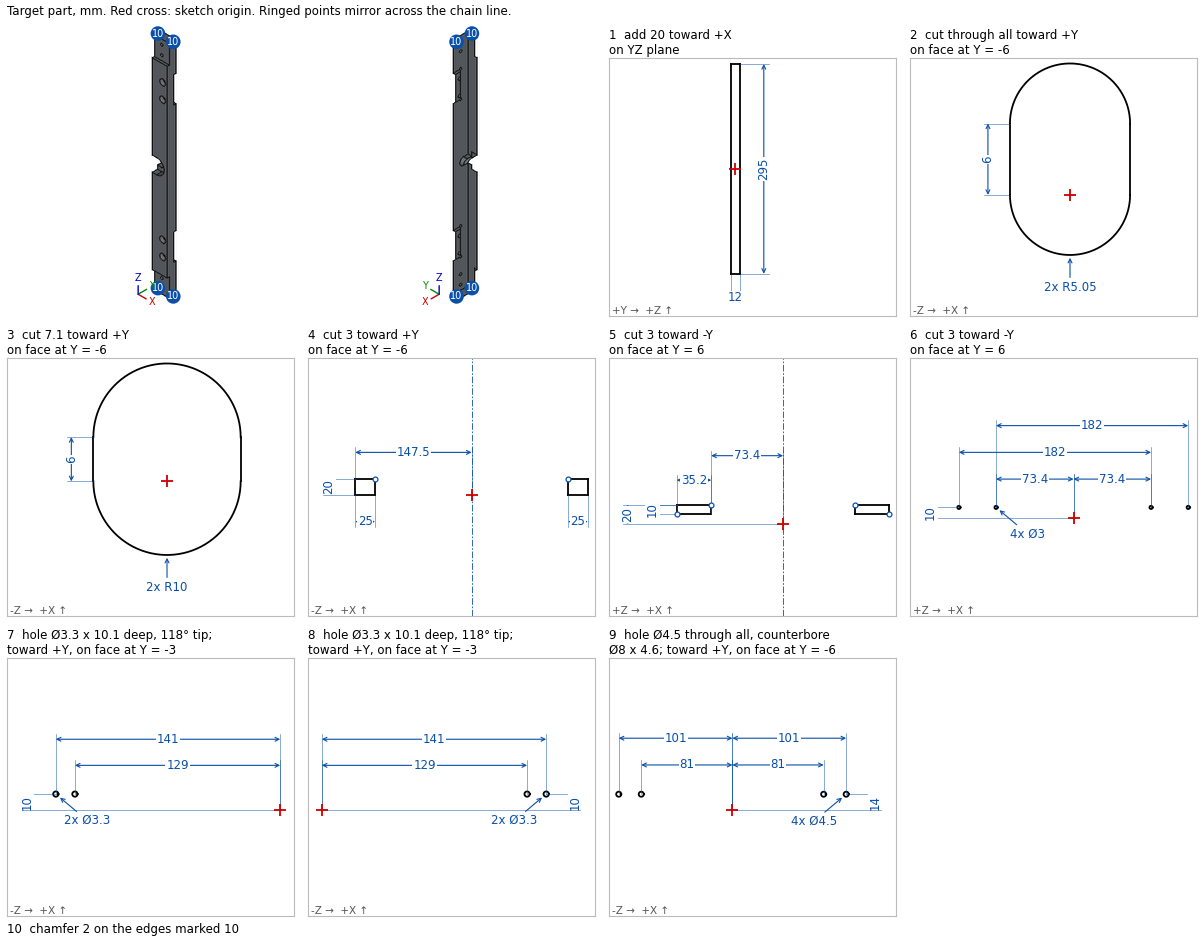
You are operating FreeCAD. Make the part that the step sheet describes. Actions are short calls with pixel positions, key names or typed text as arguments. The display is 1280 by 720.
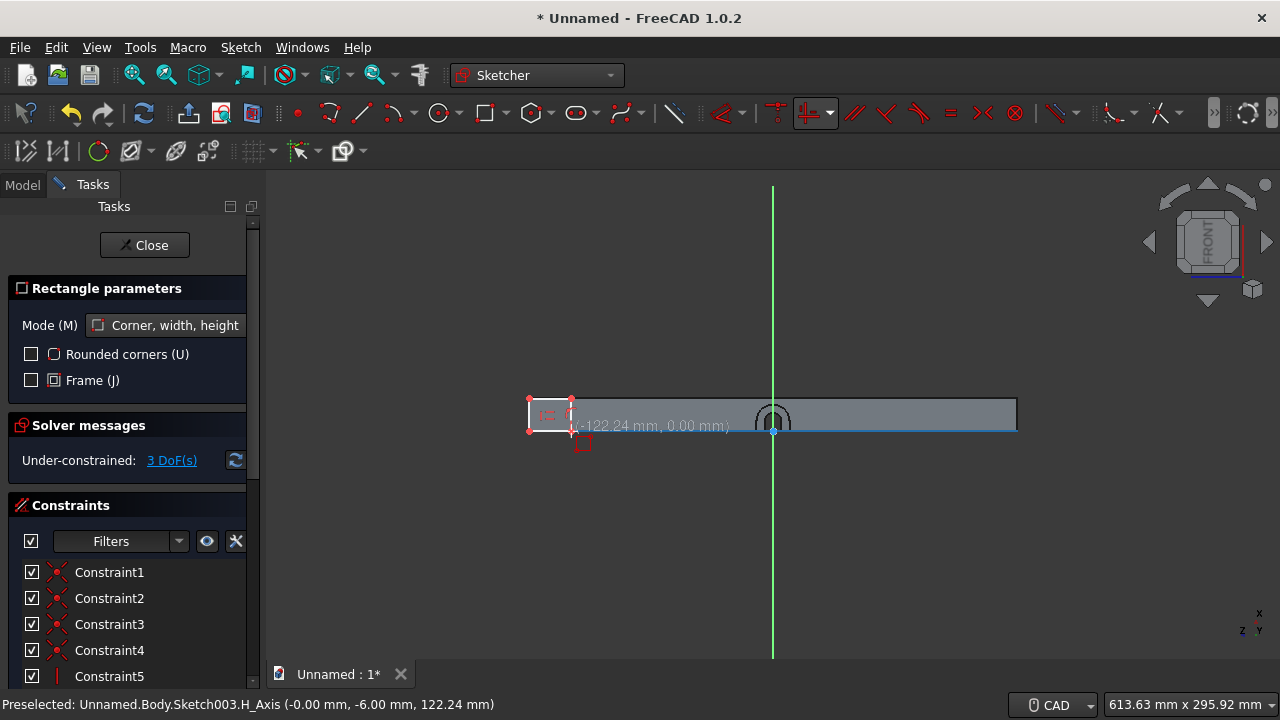
click(975, 398)
click(1017, 431)
key(Escape)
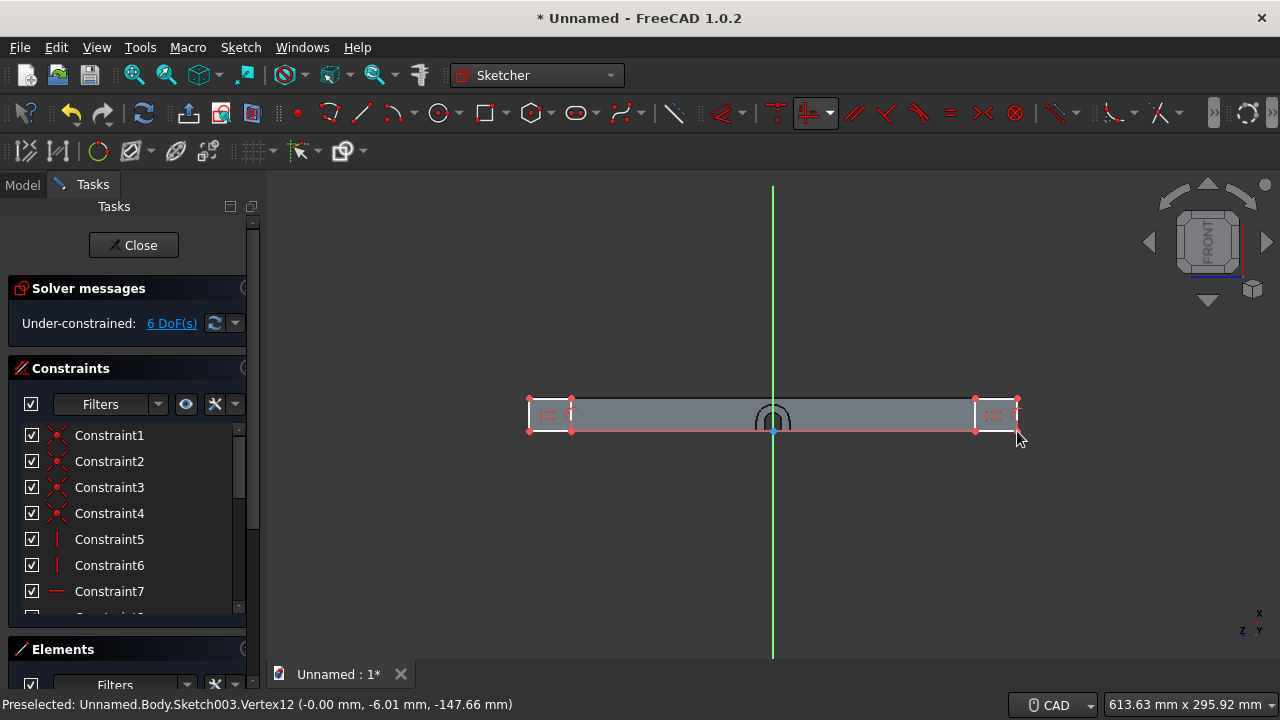
click(571, 399)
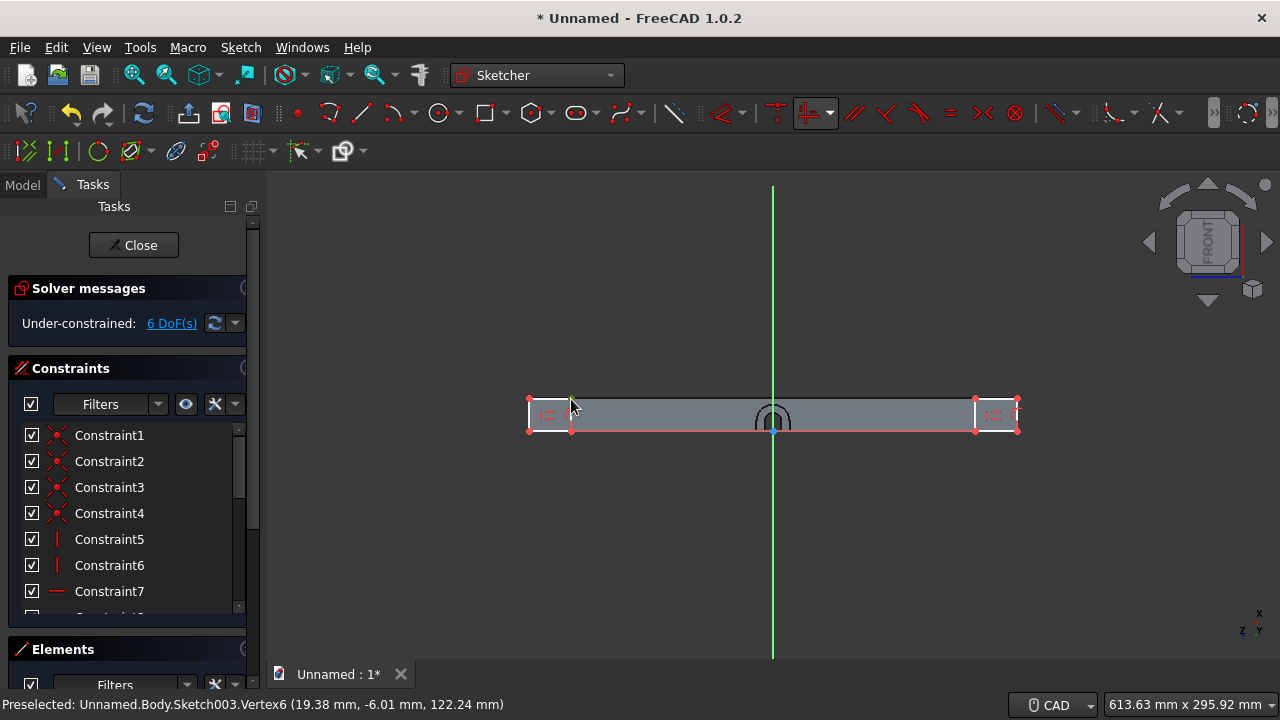
click(975, 399)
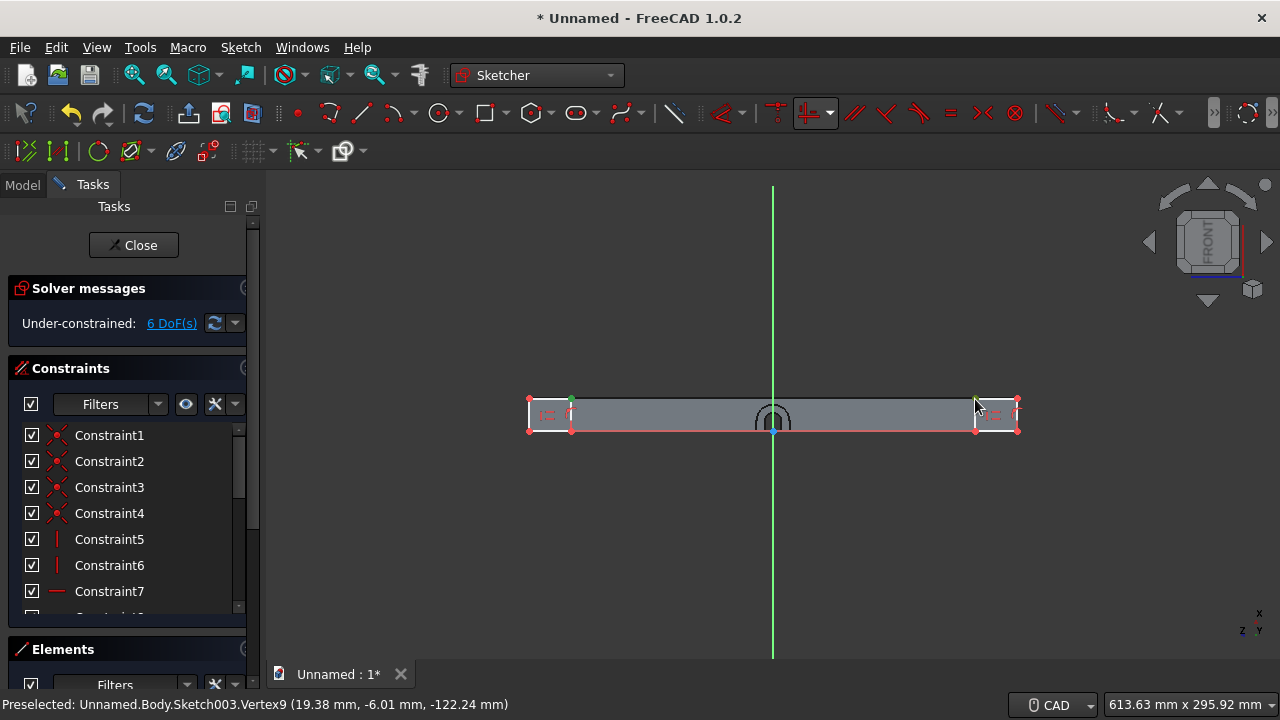
click(773, 600)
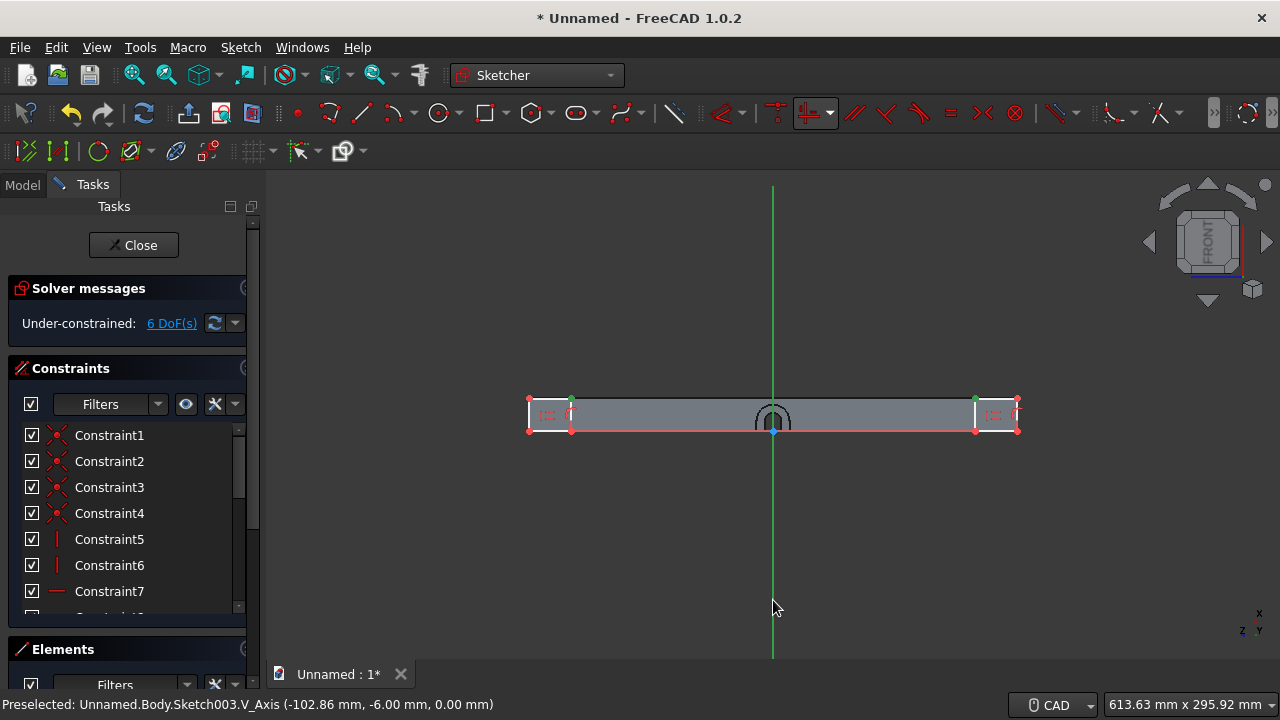
click(984, 114)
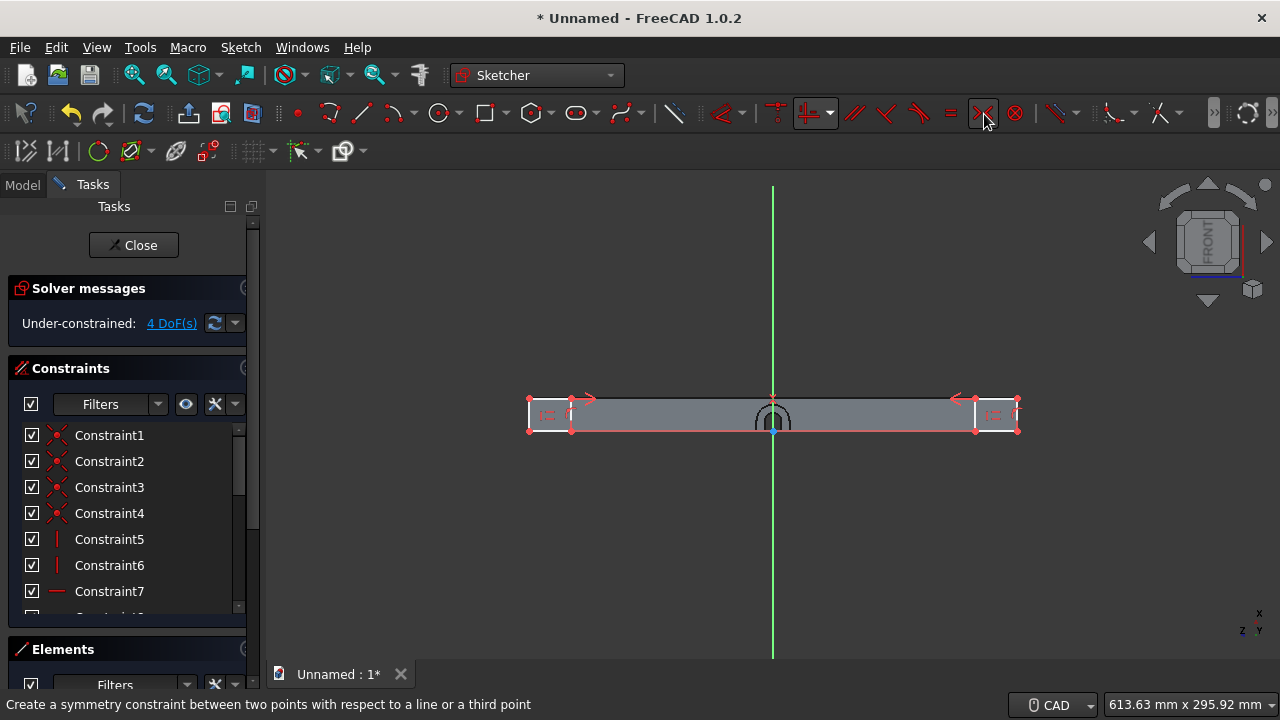
click(722, 114)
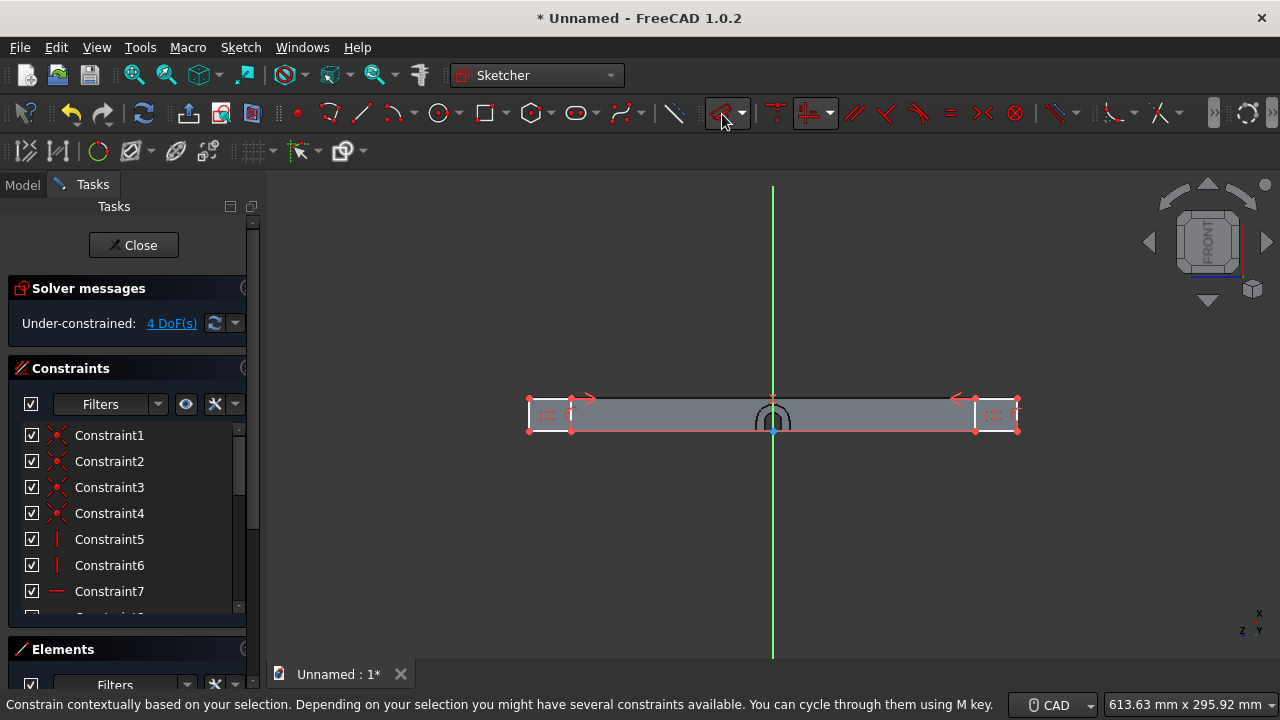
scroll(529, 409, up, 2)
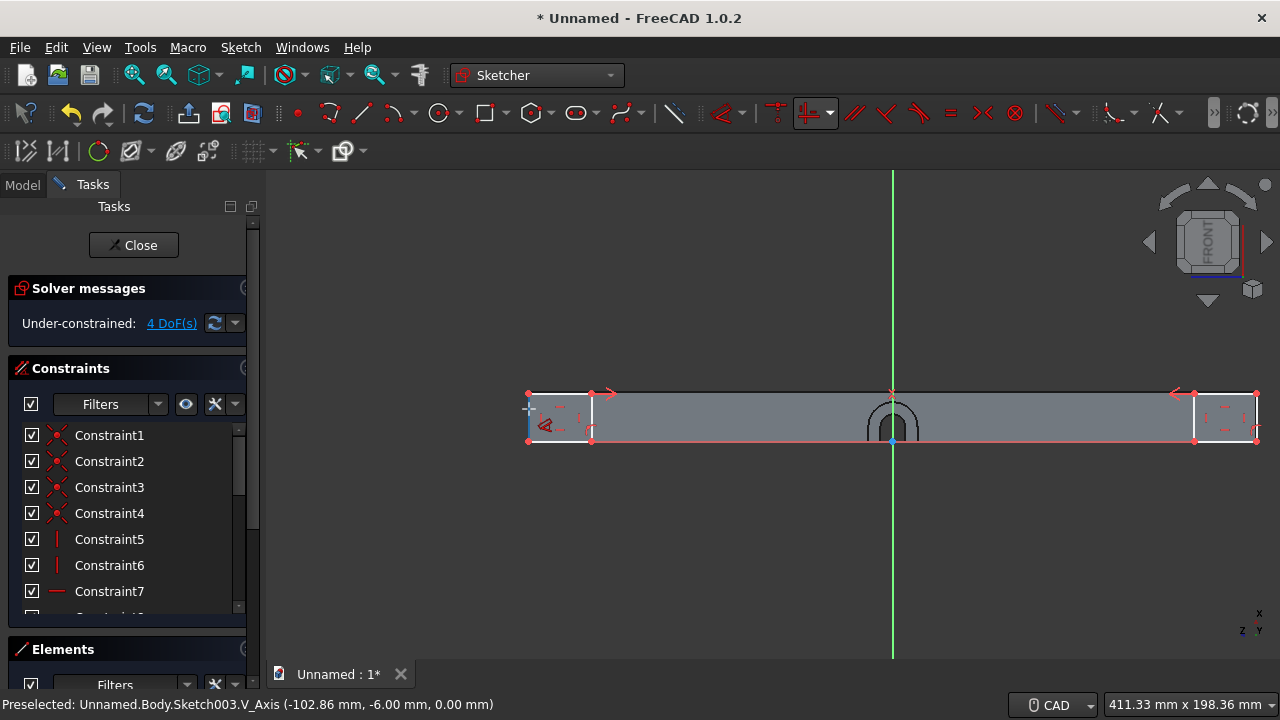
click(529, 408)
click(495, 418)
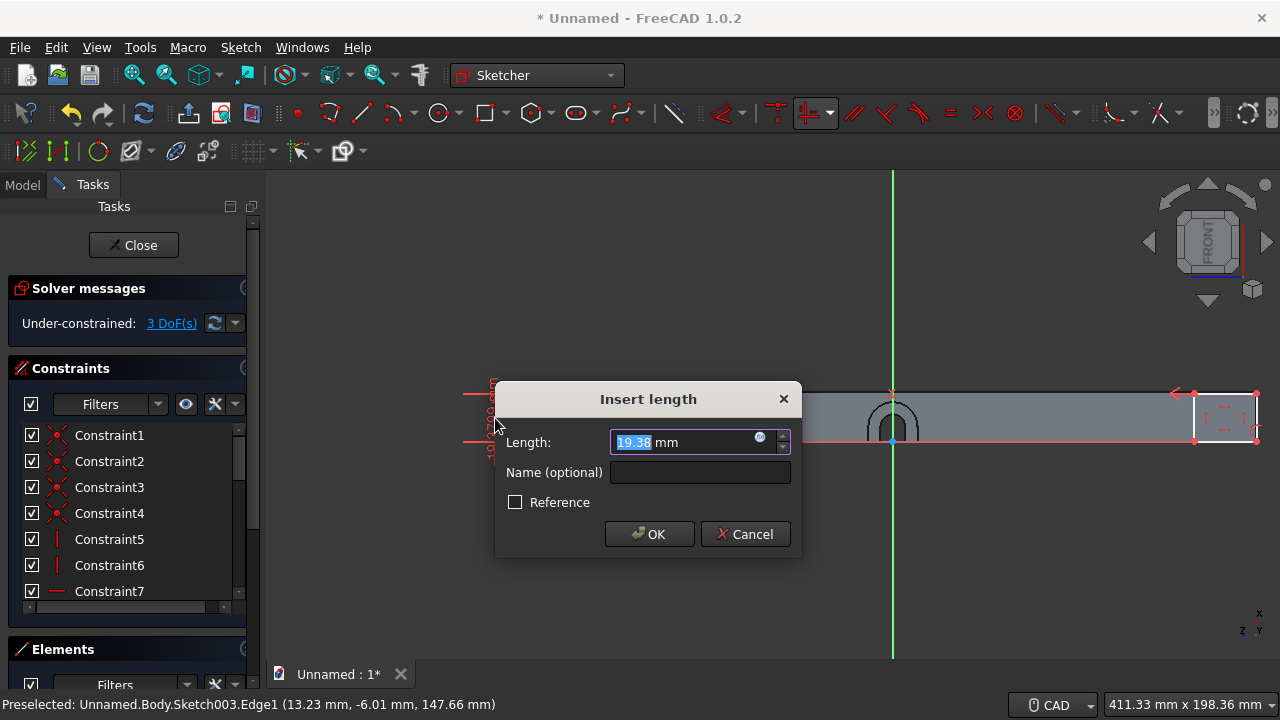
text(20)
key(Return)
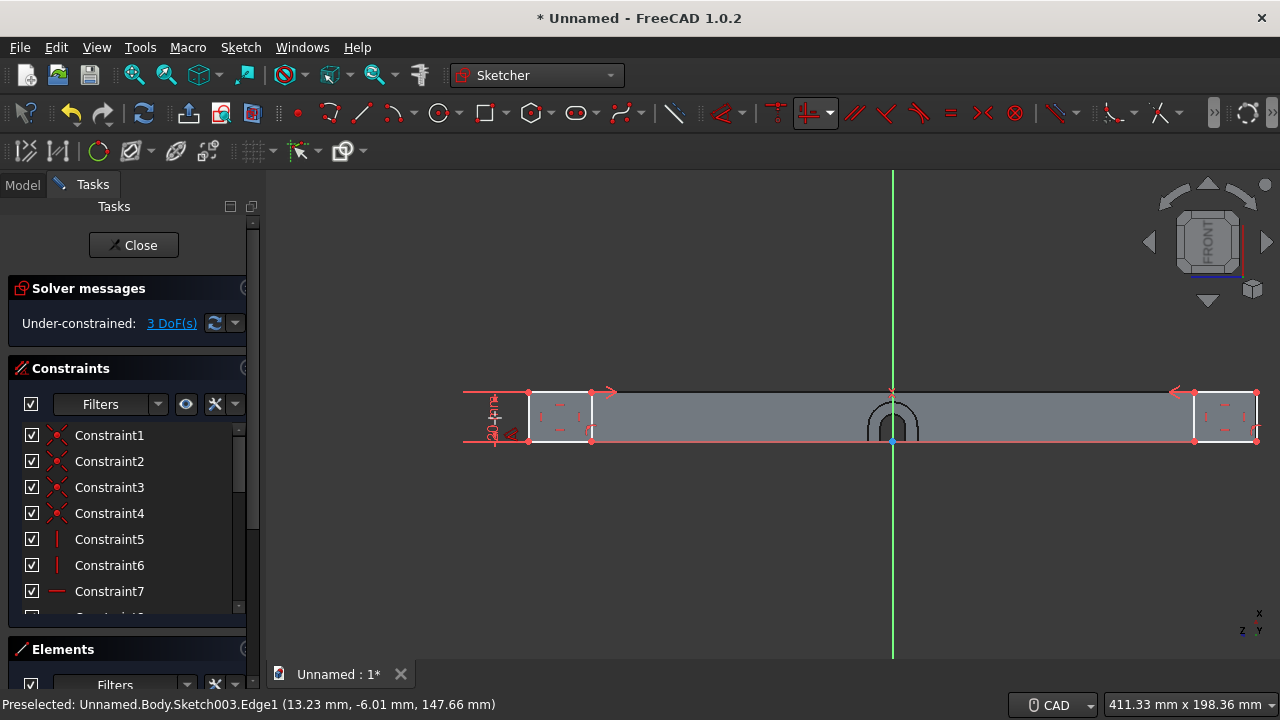
click(548, 442)
click(560, 476)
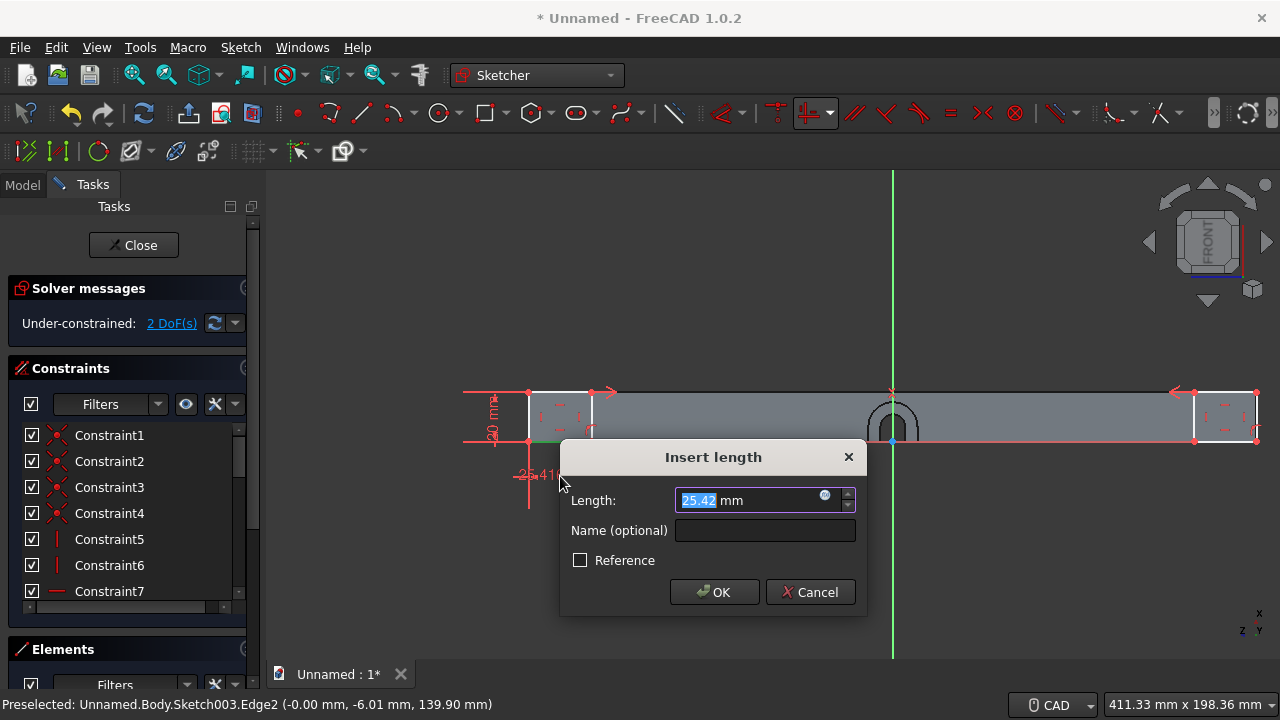
text(25)
key(Return)